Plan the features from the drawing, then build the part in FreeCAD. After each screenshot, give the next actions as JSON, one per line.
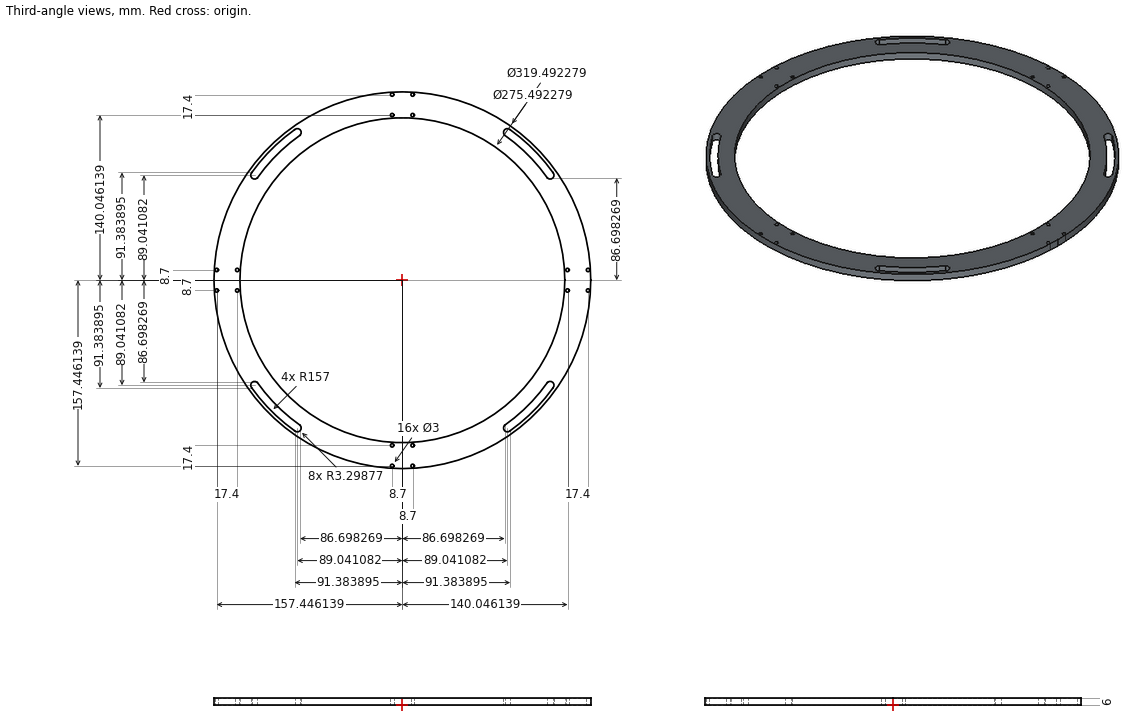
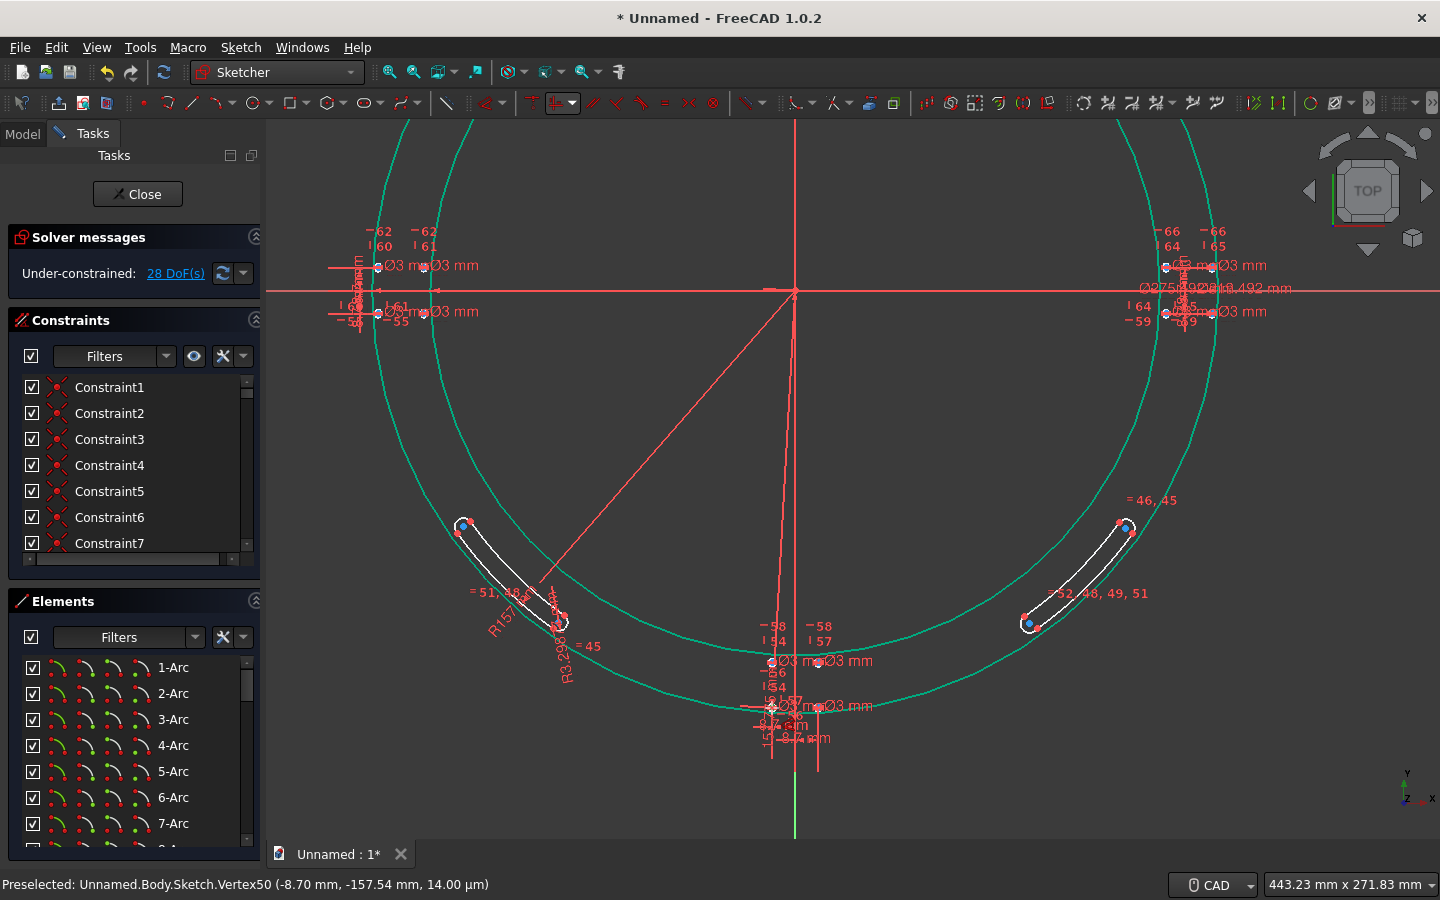
{"action": "left_click", "coordinate": [772, 663]}
{"action": "left_click", "coordinate": [738, 685]}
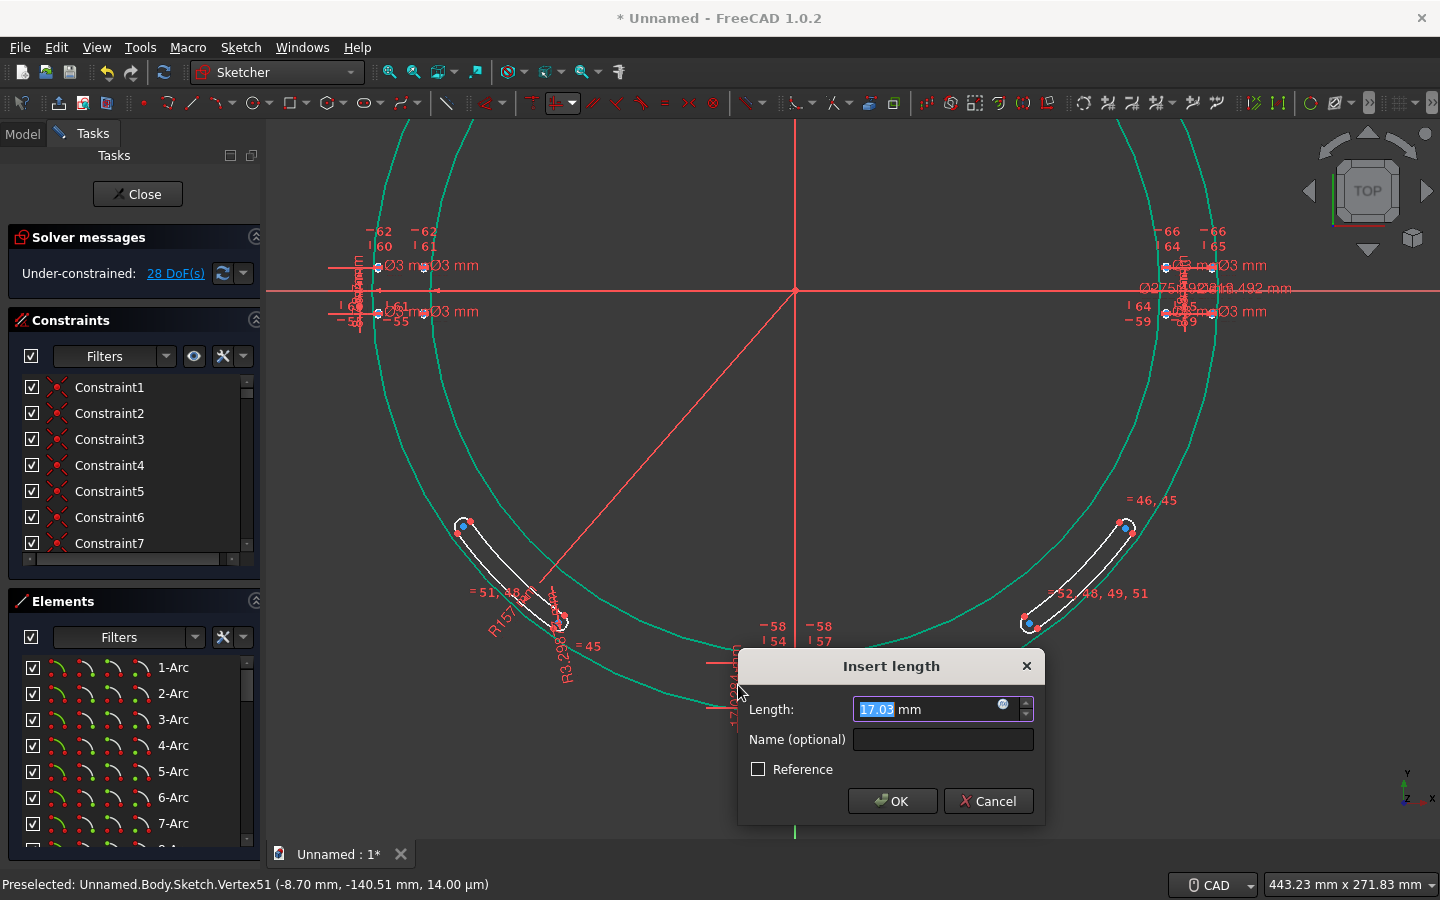
{"action": "type", "text": "17.4"}
{"action": "key", "text": "Return"}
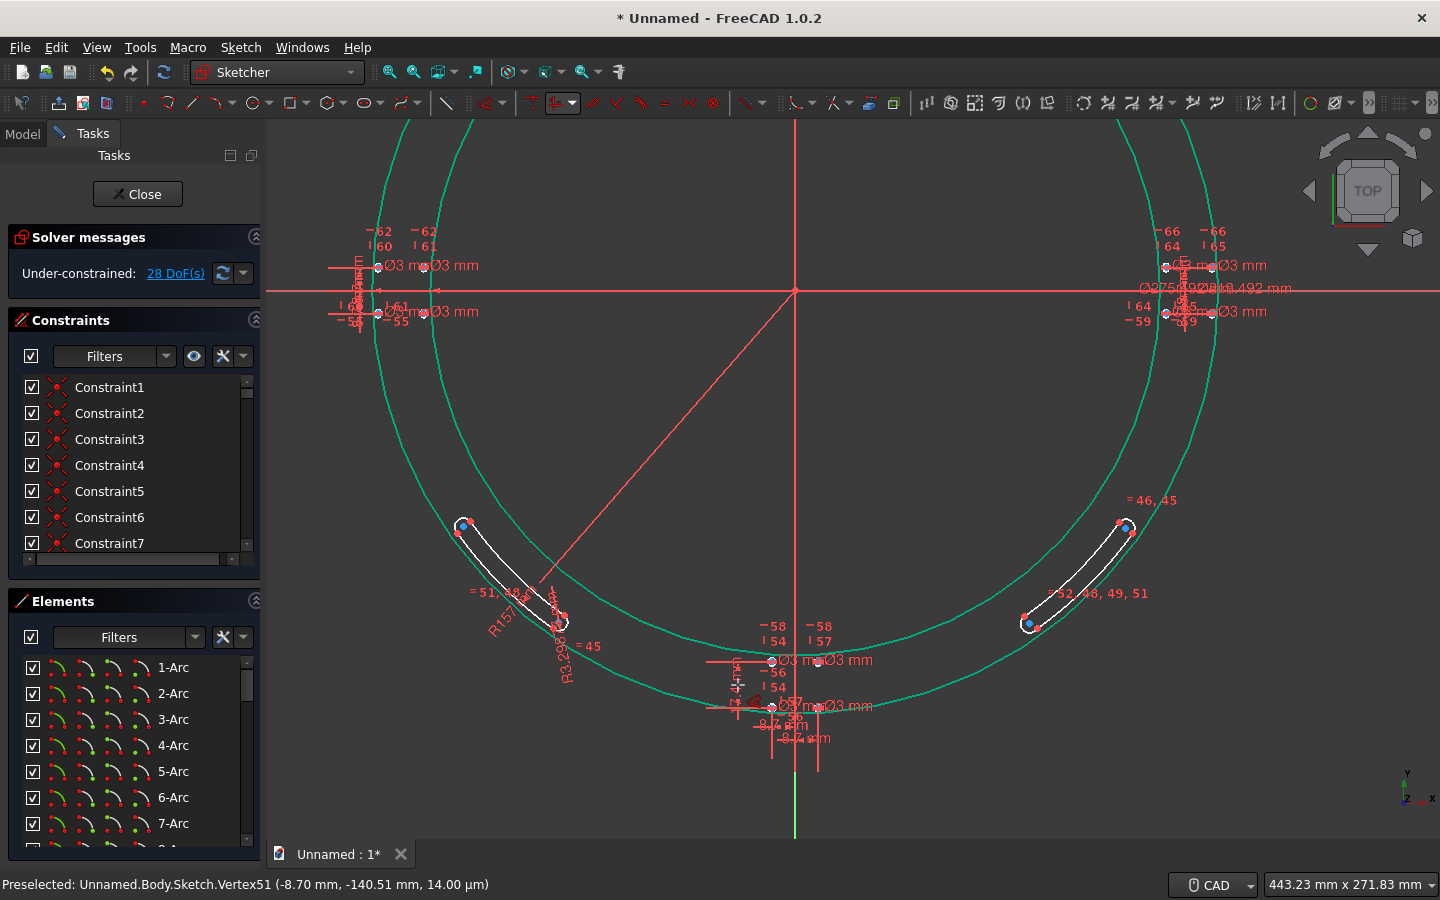
{"action": "left_click", "coordinate": [378, 314]}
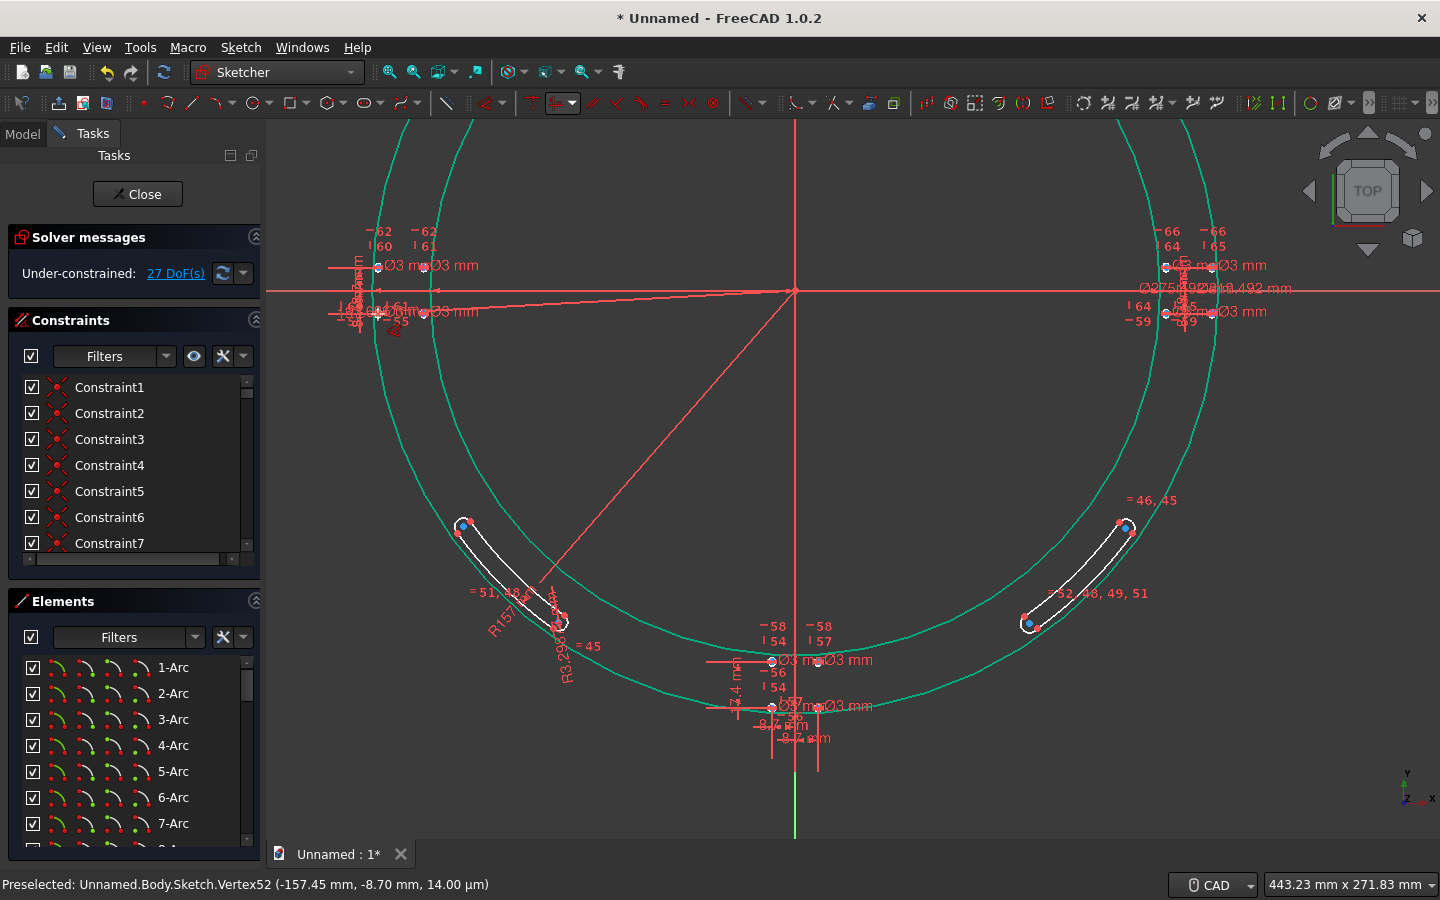
{"action": "left_click", "coordinate": [424, 314]}
{"action": "left_click", "coordinate": [401, 348]}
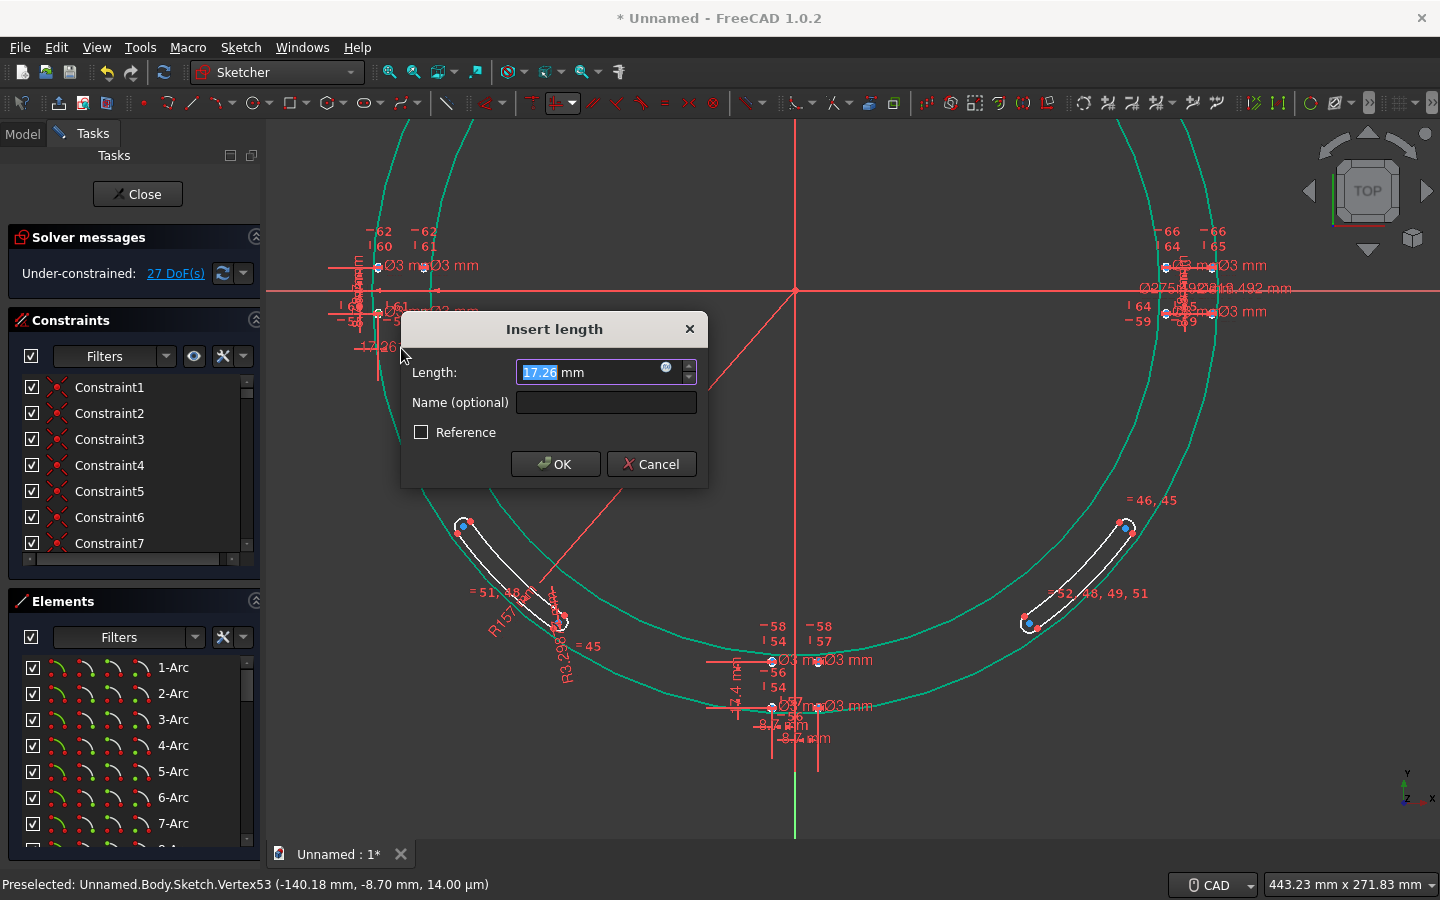
{"action": "type", "text": "17.4"}
{"action": "key", "text": "Return"}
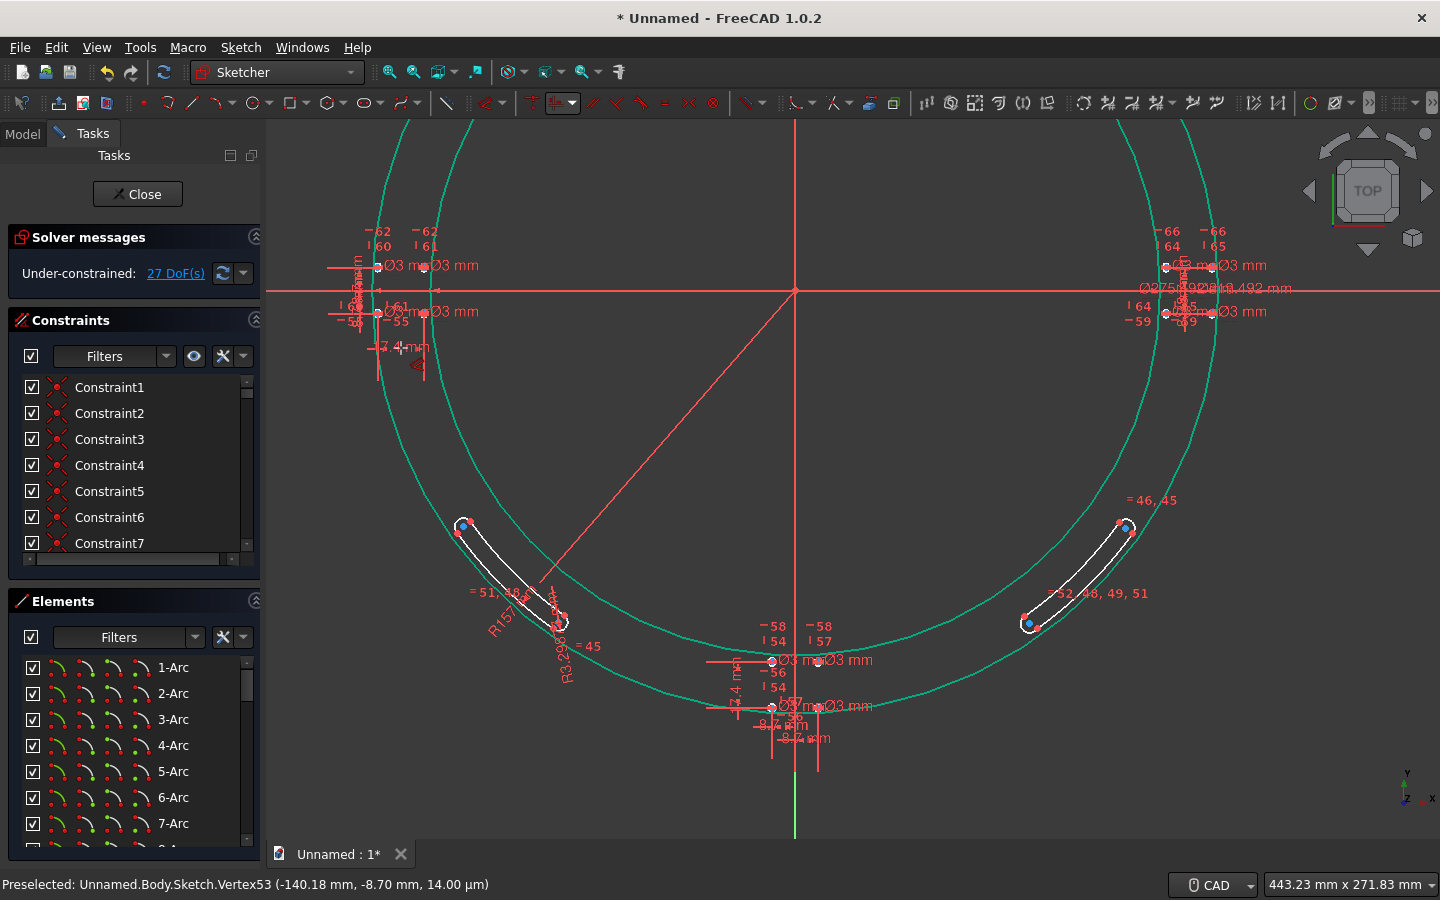
{"action": "left_click", "coordinate": [1166, 314]}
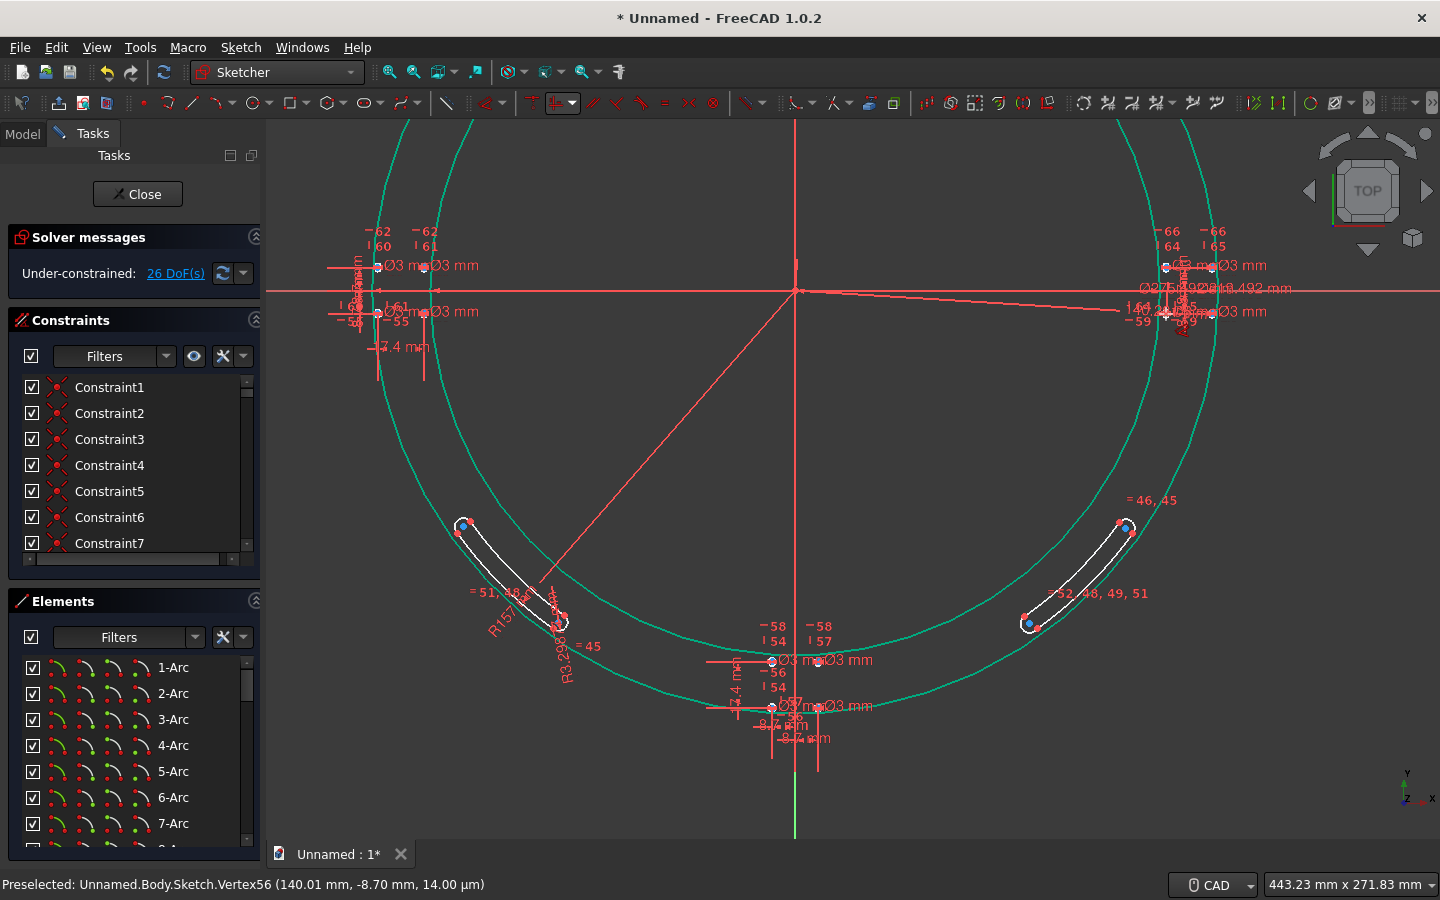
{"action": "left_click", "coordinate": [1212, 314]}
{"action": "left_click", "coordinate": [1189, 348]}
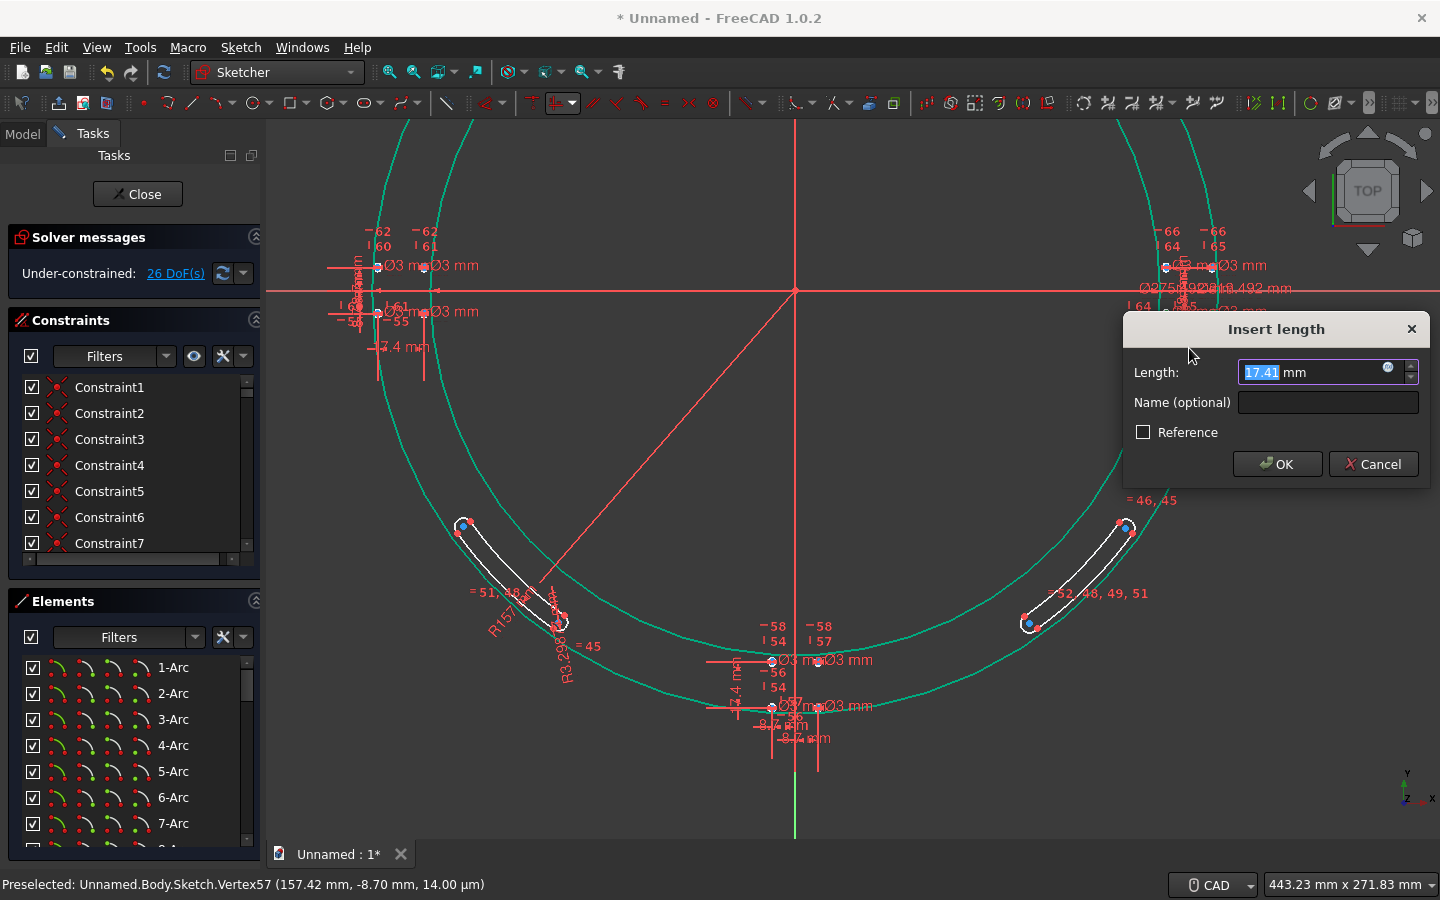
{"action": "type", "text": "17.4"}
{"action": "key", "text": "Return"}